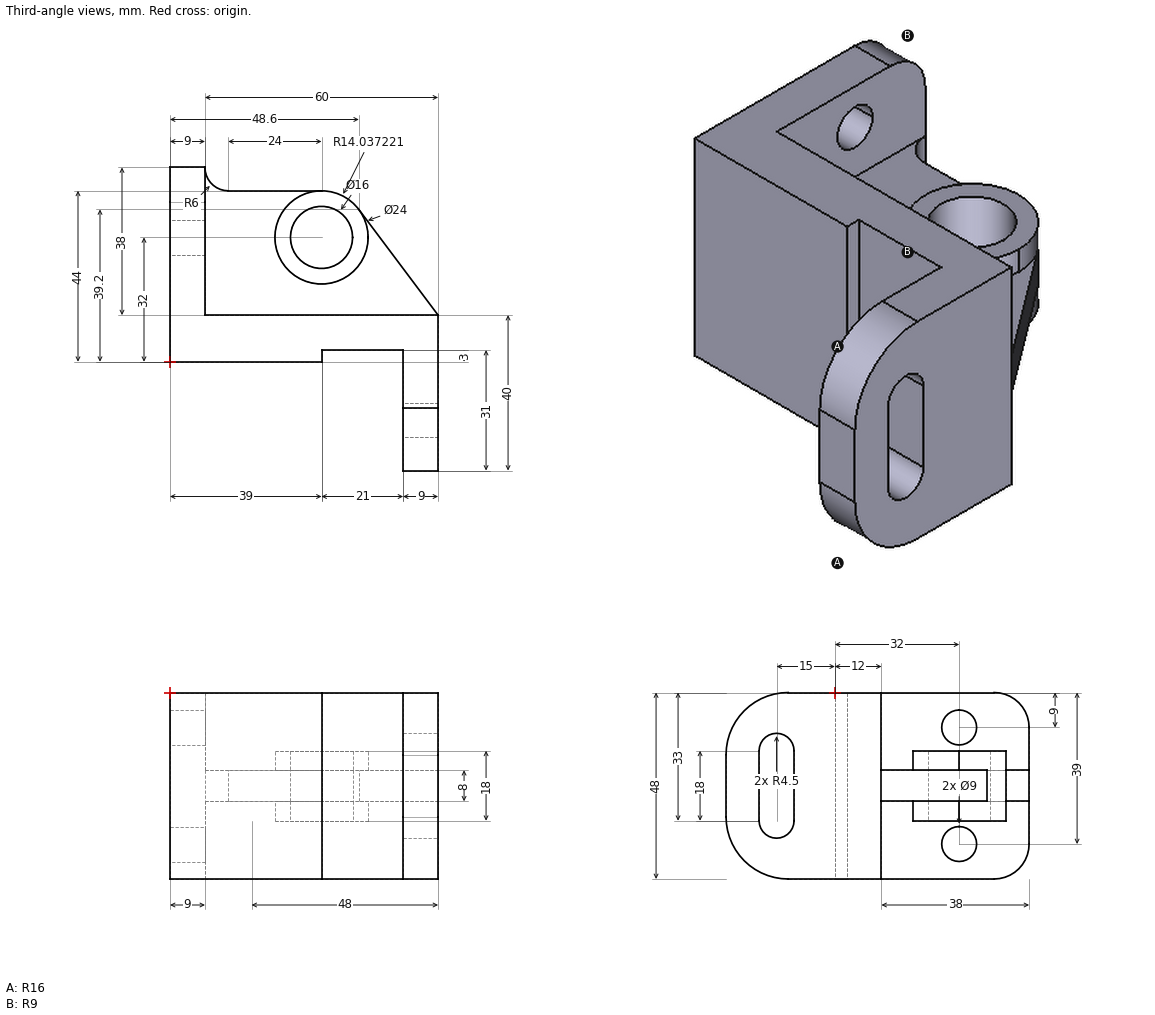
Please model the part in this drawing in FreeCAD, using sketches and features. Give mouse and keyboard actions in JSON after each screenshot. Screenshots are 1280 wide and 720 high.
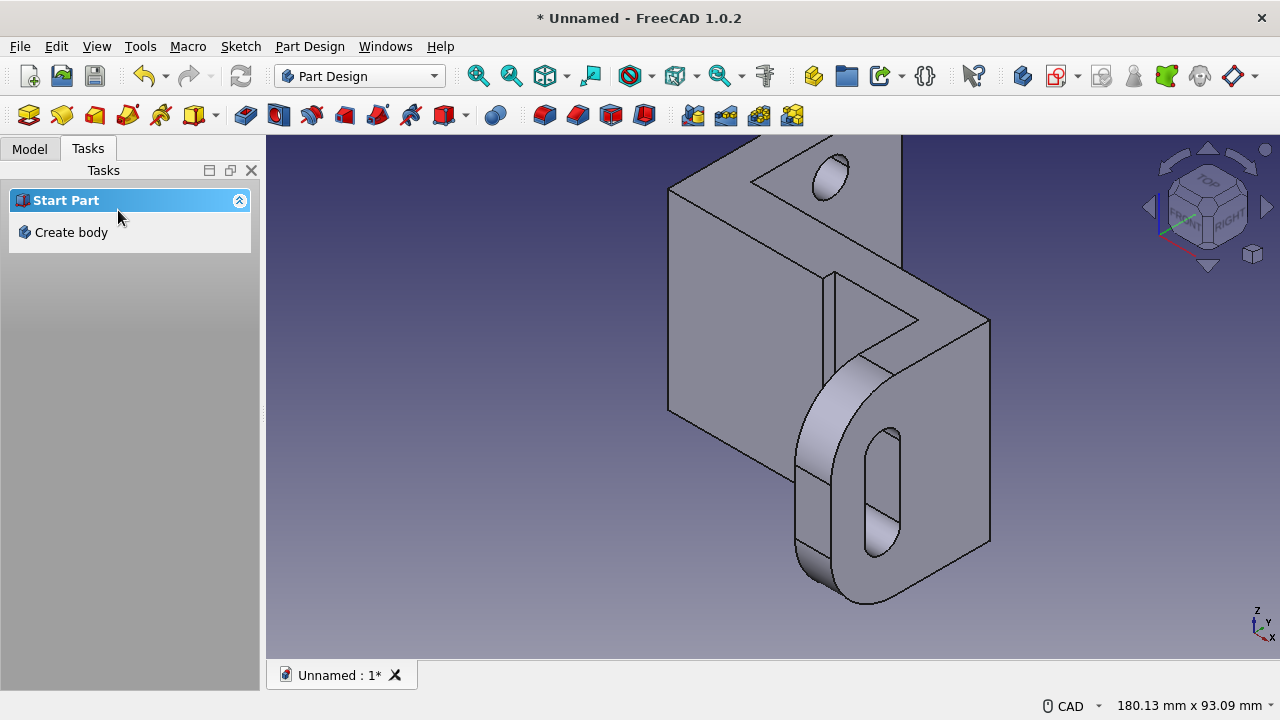
{"action": "key", "text": "v f"}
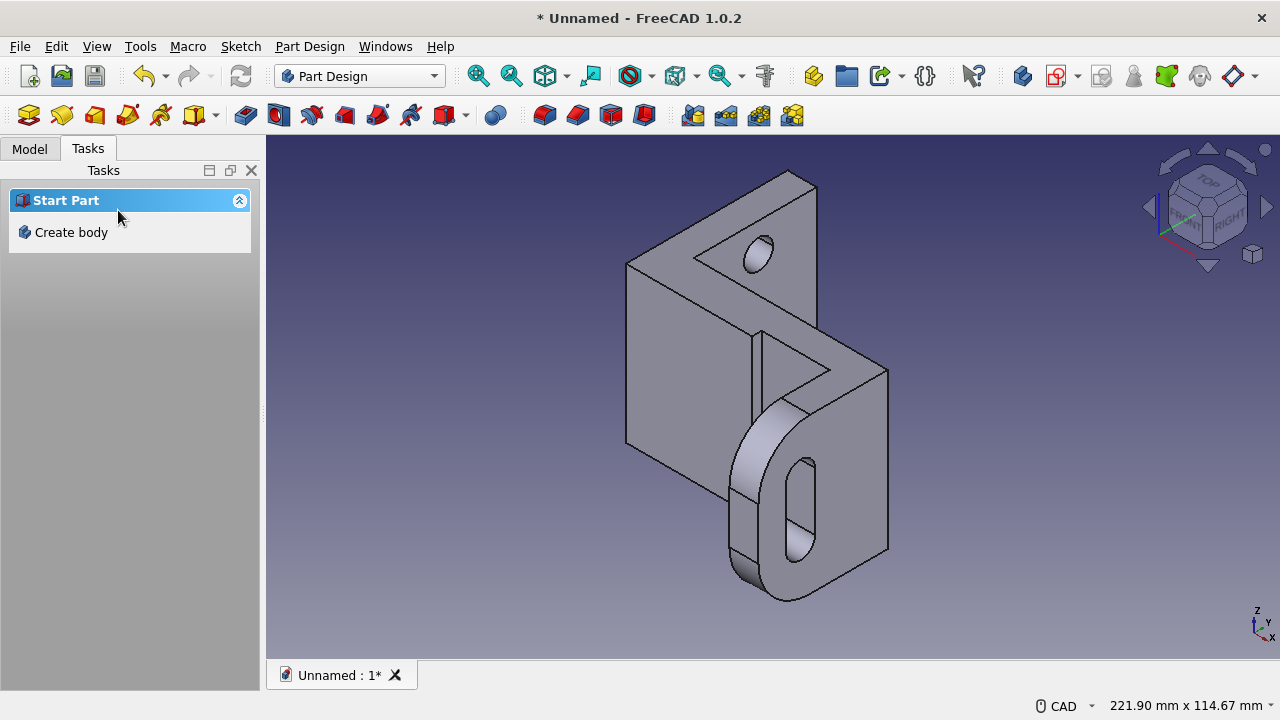
{"action": "left_click", "coordinate": [1023, 76]}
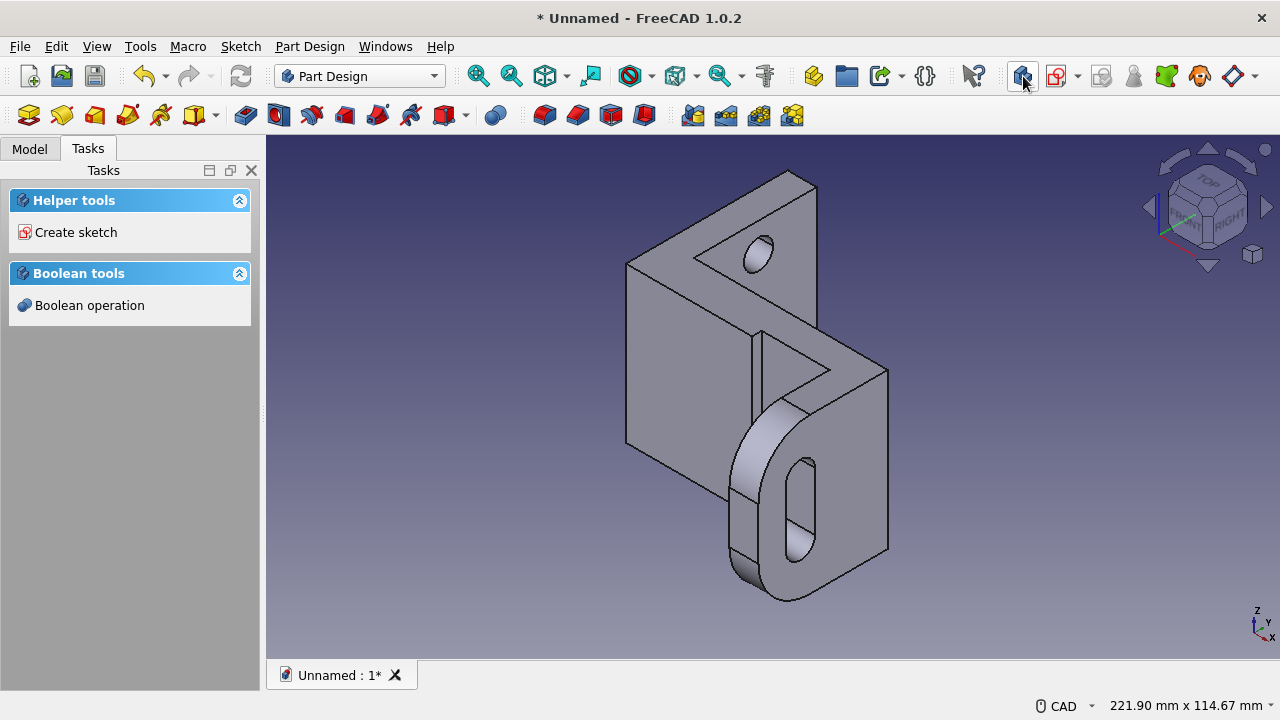
{"action": "left_click", "coordinate": [30, 148]}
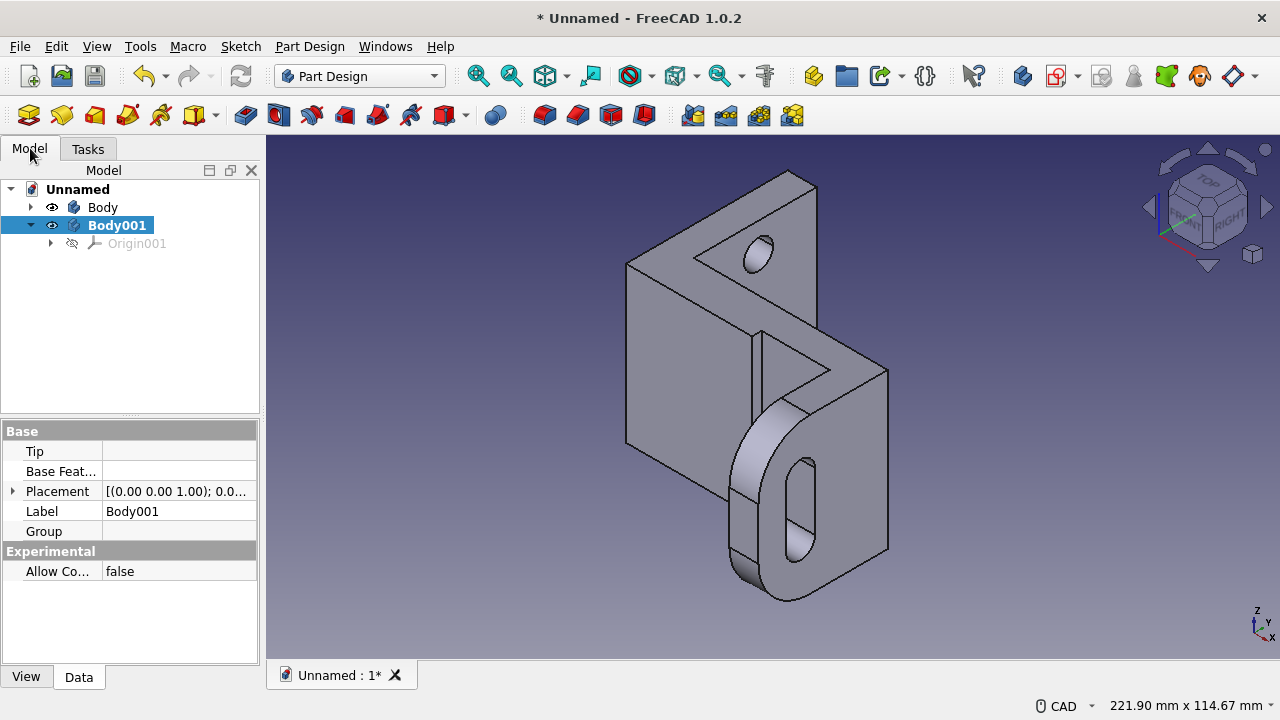
{"action": "left_click", "coordinate": [51, 243]}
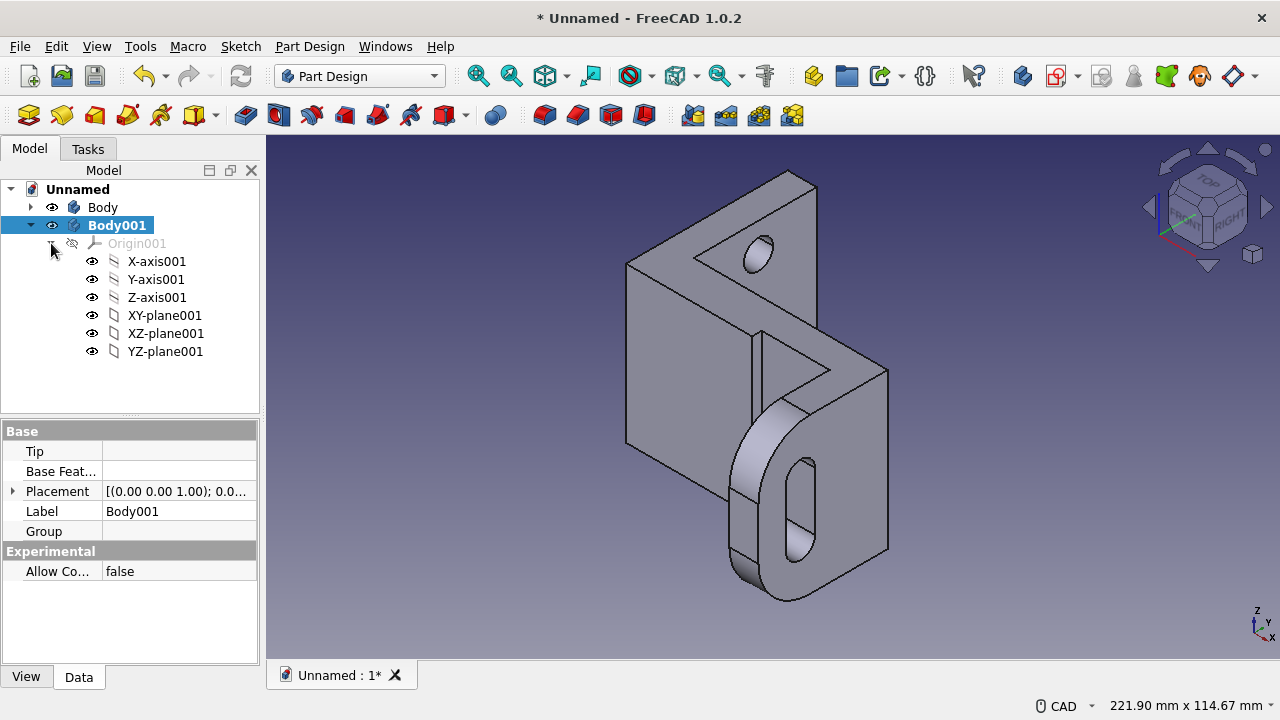
{"action": "left_click", "coordinate": [137, 315]}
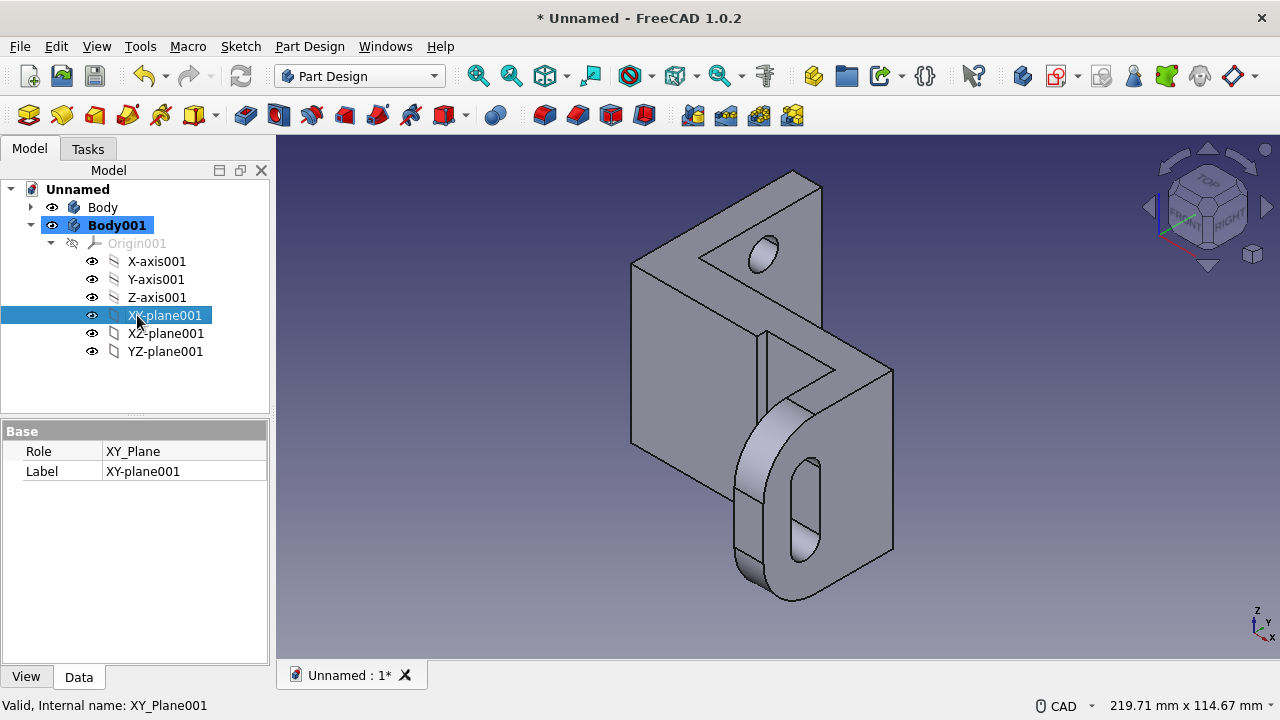
{"action": "left_click", "coordinate": [1232, 76]}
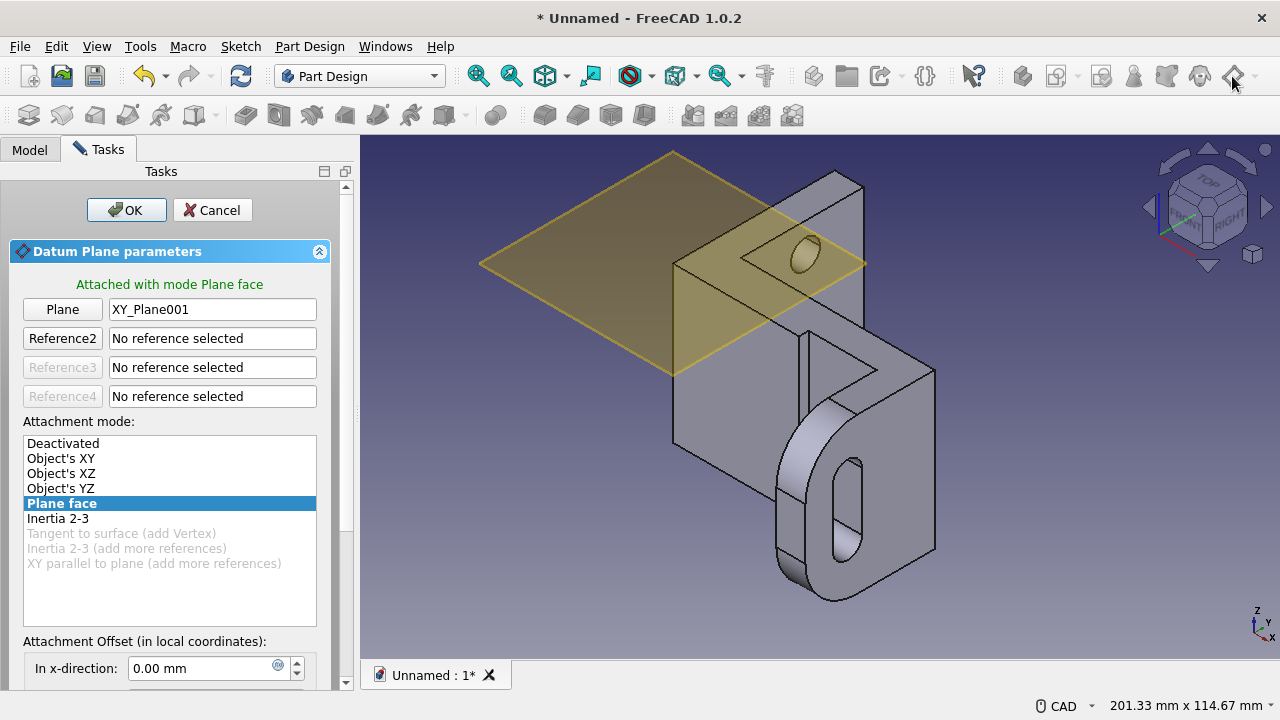
{"action": "scroll", "coordinate": [346, 436], "scroll_direction": "down", "scroll_amount": 2}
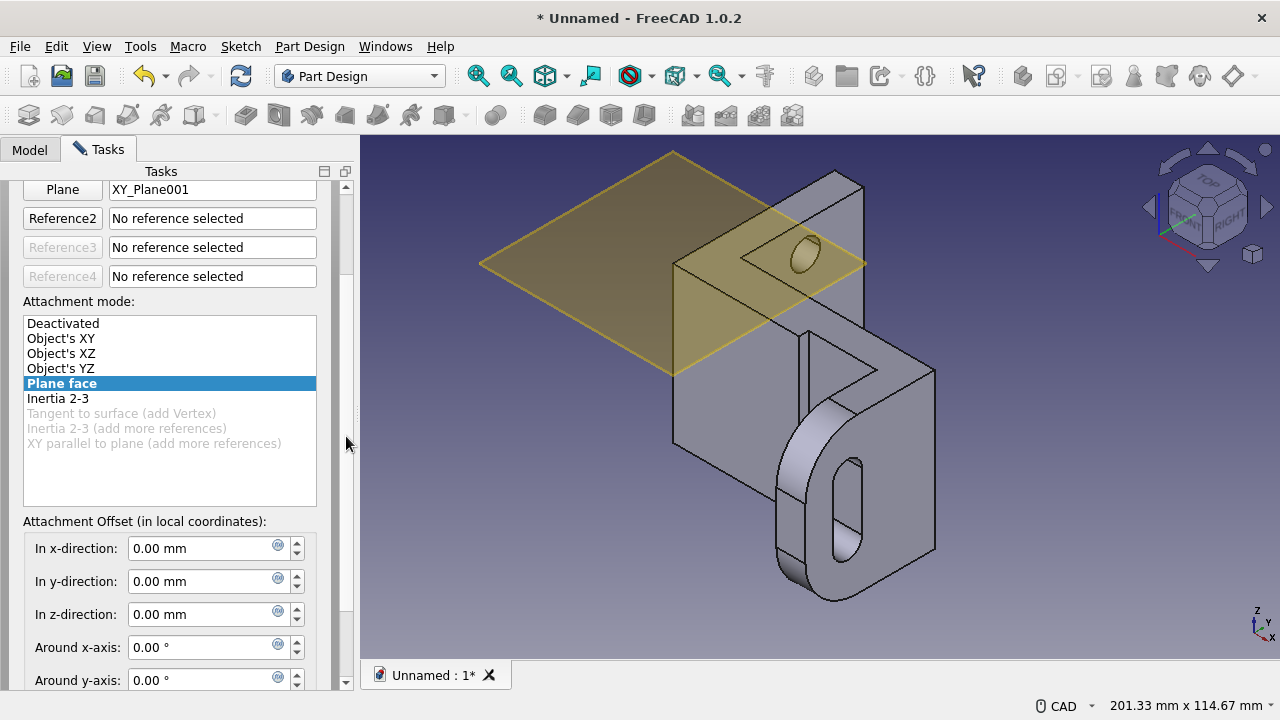
{"action": "triple_click", "coordinate": [210, 614]}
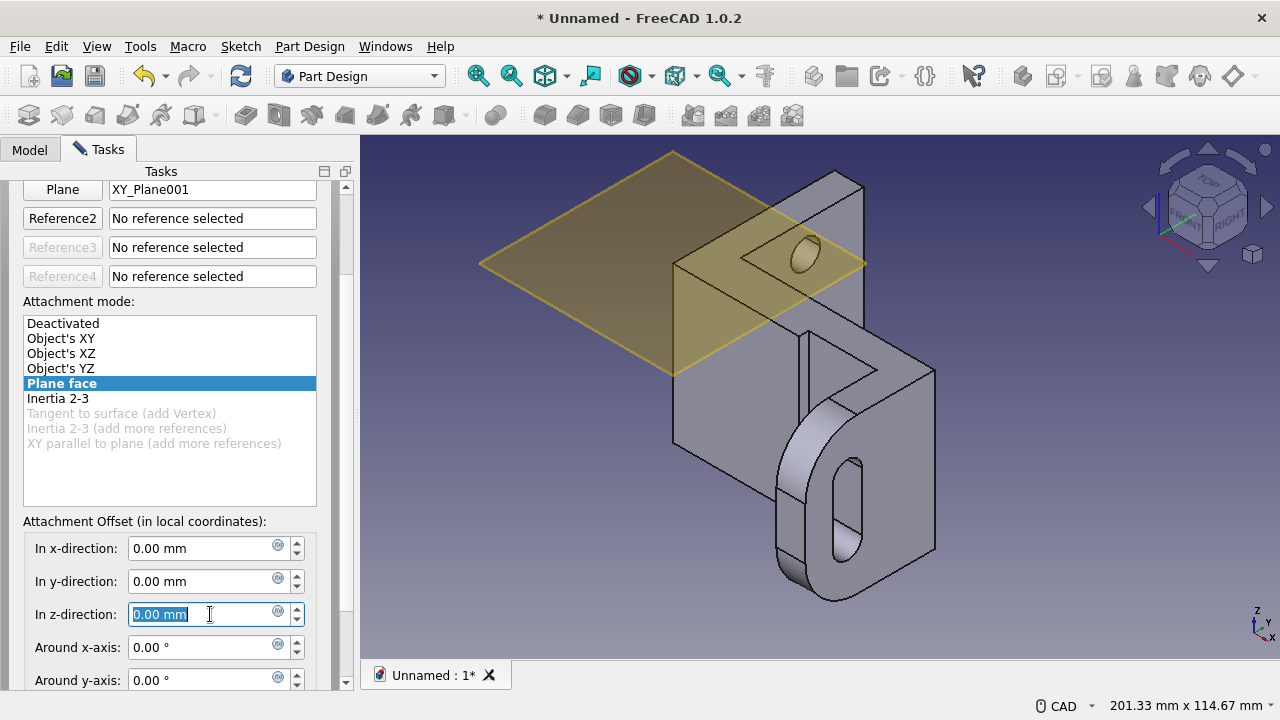
{"action": "type", "text": "-24"}
{"action": "key", "text": "Tab"}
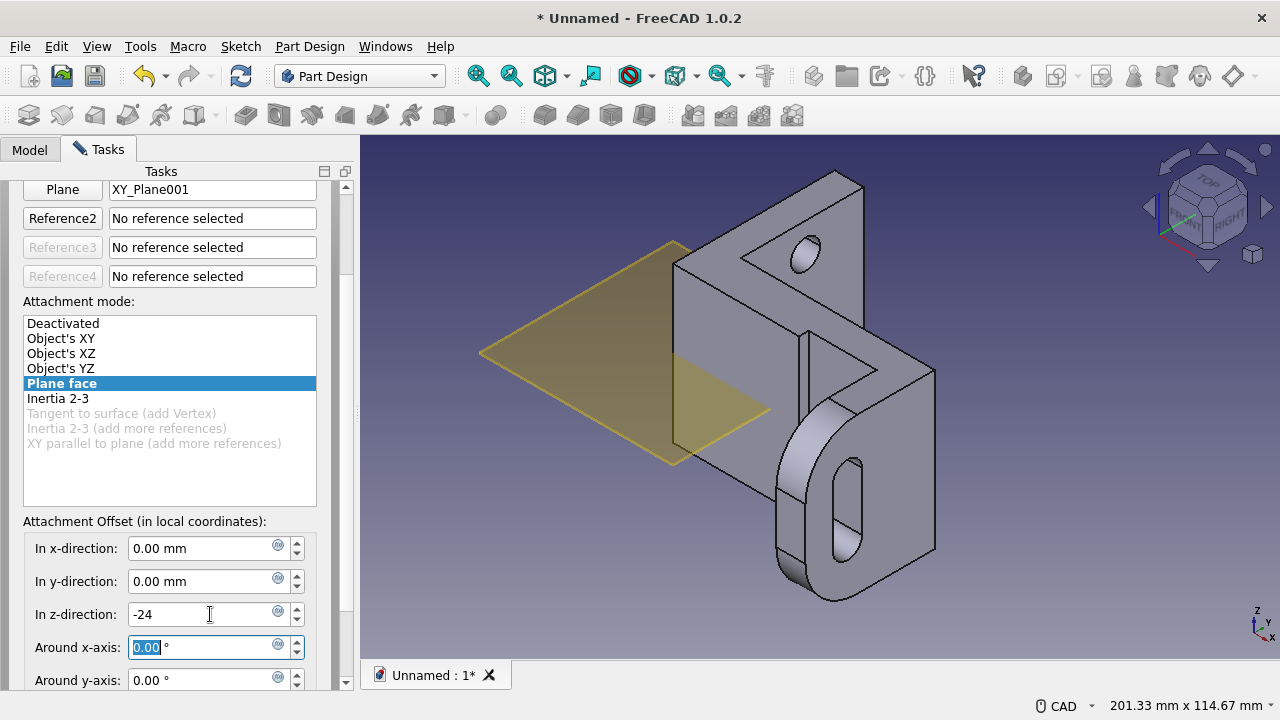
{"action": "scroll", "coordinate": [346, 436], "scroll_direction": "up", "scroll_amount": 3}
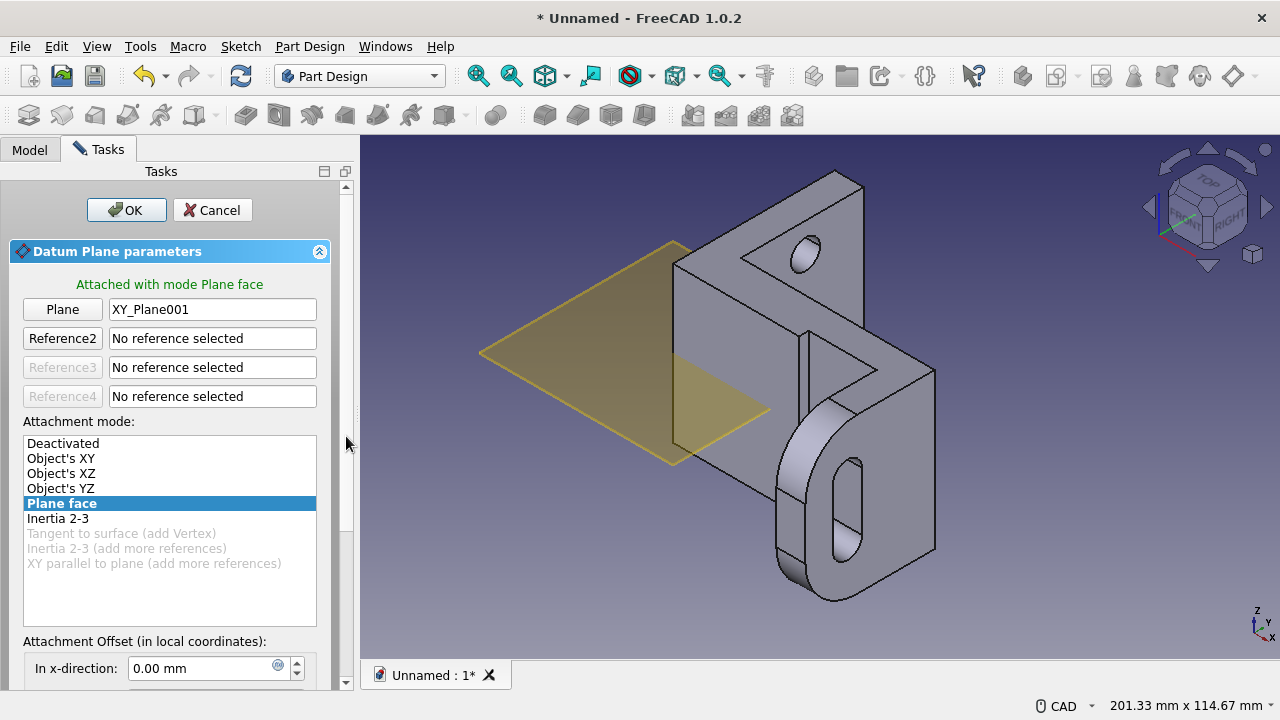
{"action": "left_click", "coordinate": [127, 210]}